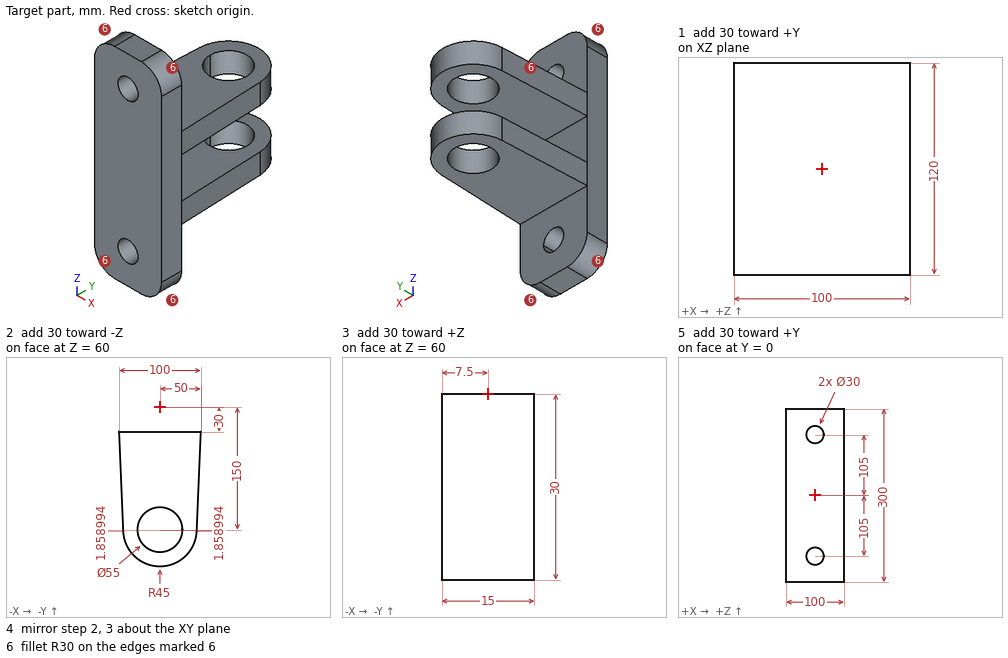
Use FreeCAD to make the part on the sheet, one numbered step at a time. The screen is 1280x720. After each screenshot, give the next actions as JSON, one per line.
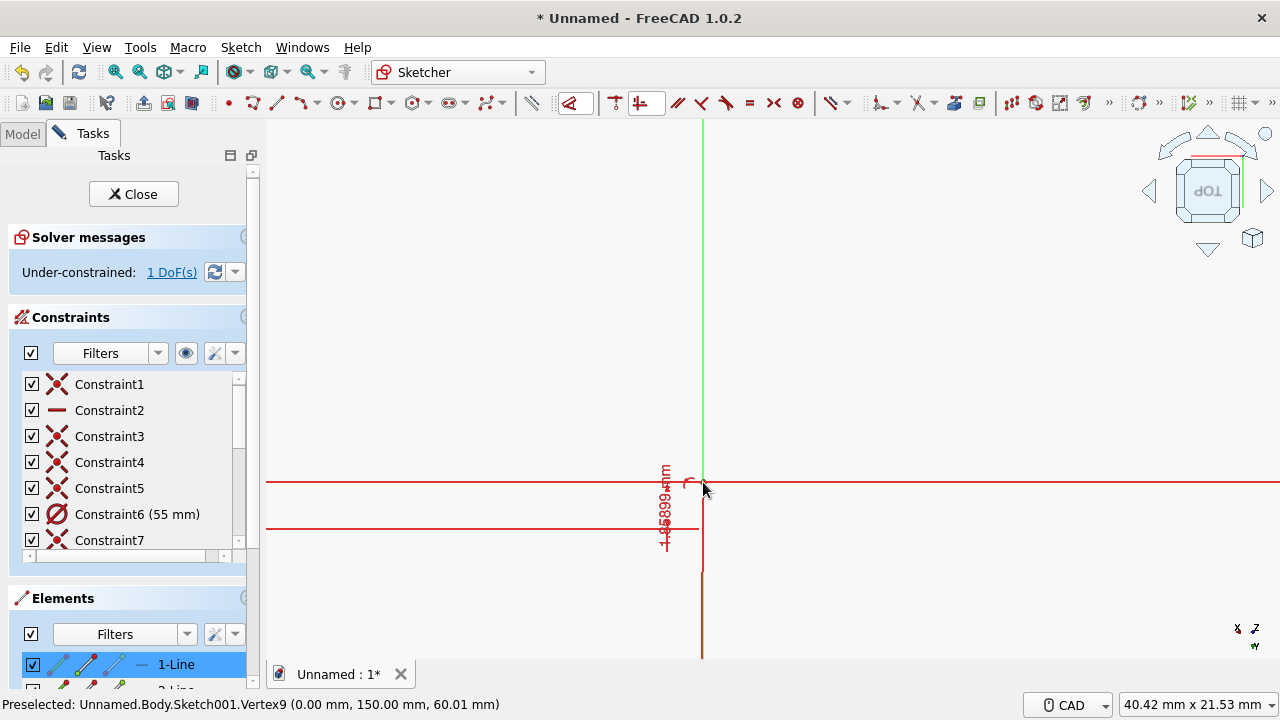
{"action": "key", "text": "i"}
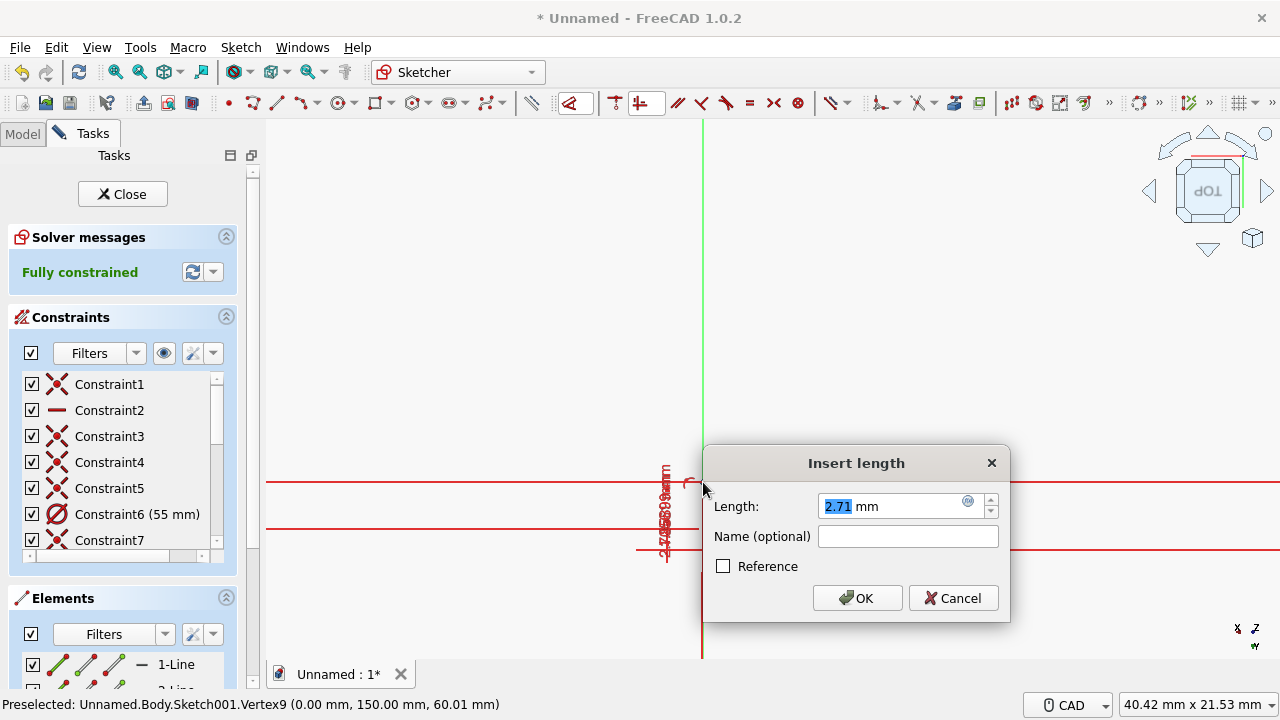
{"action": "type", "text": "1.858994"}
{"action": "key", "text": "Return"}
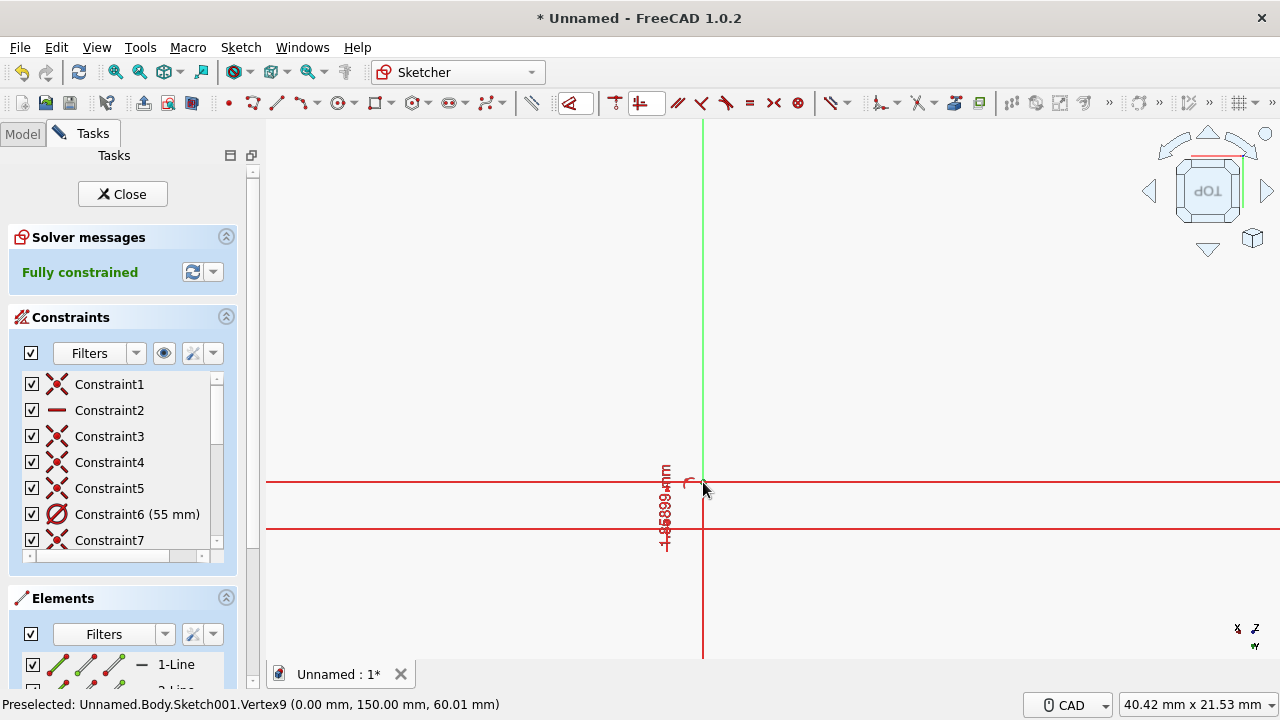
{"action": "left_click", "coordinate": [123, 194]}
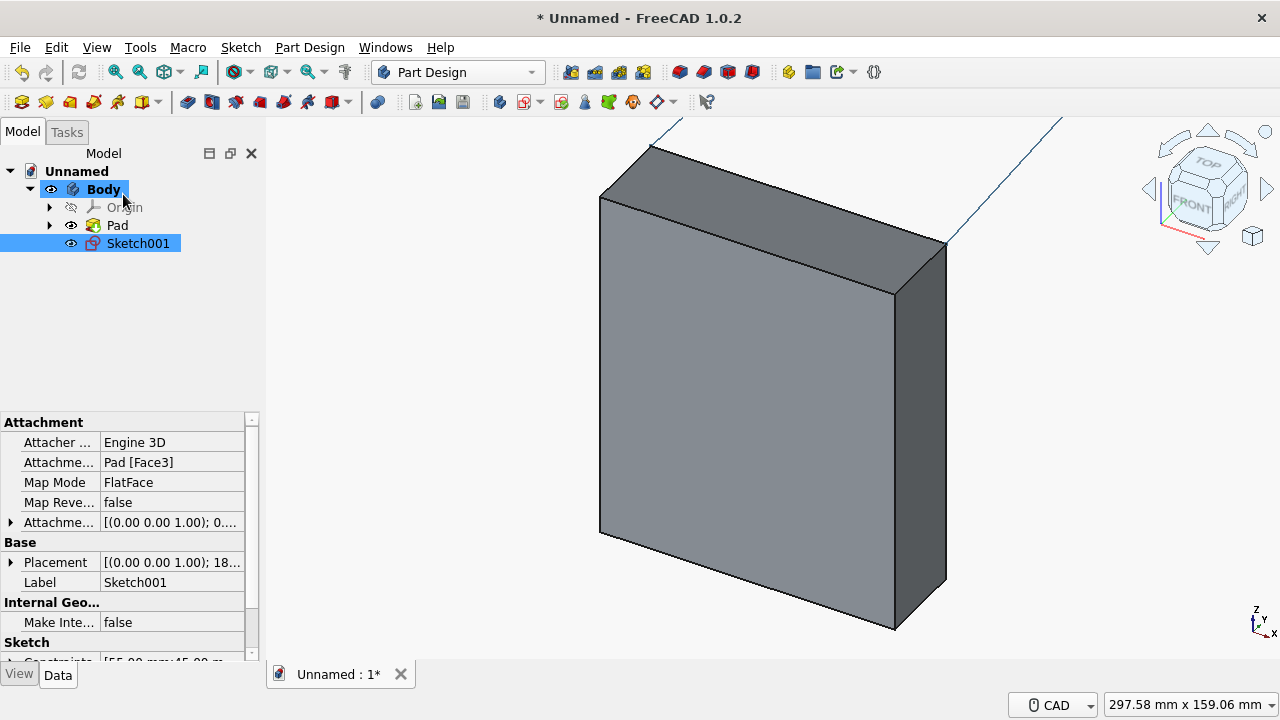
{"action": "left_click", "coordinate": [22, 102]}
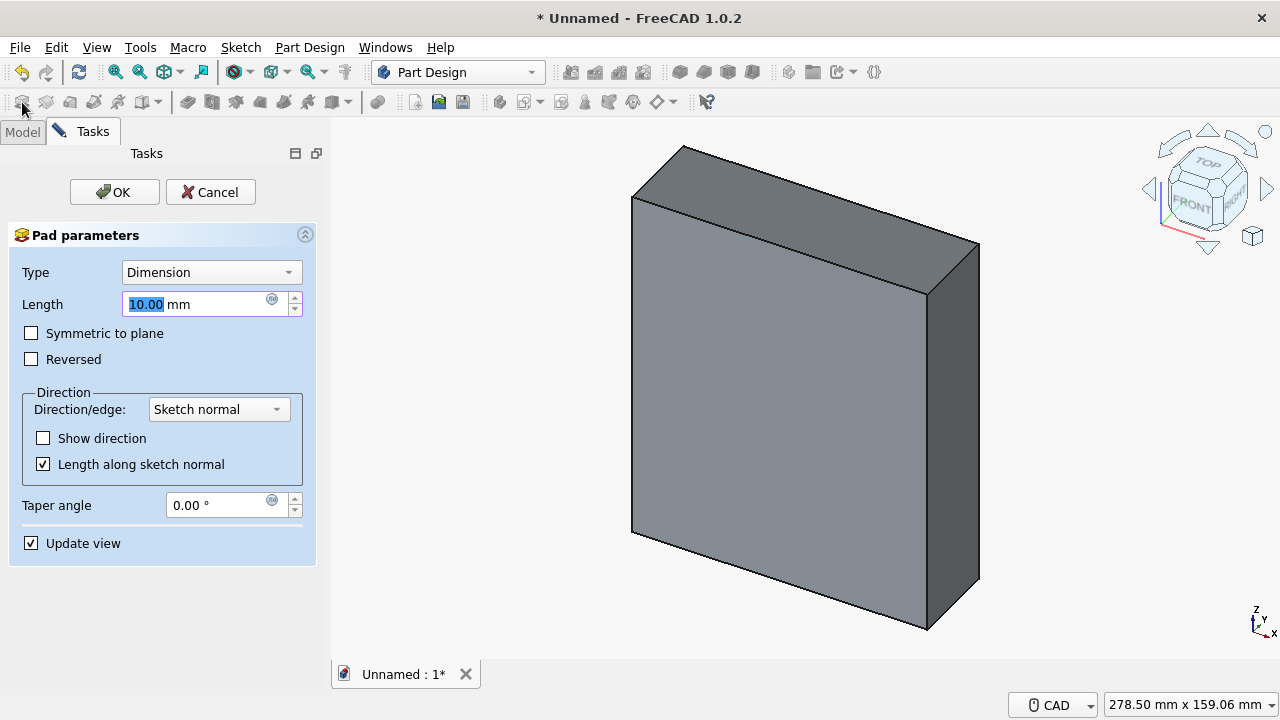
{"action": "type", "text": "30"}
{"action": "key", "text": "Tab"}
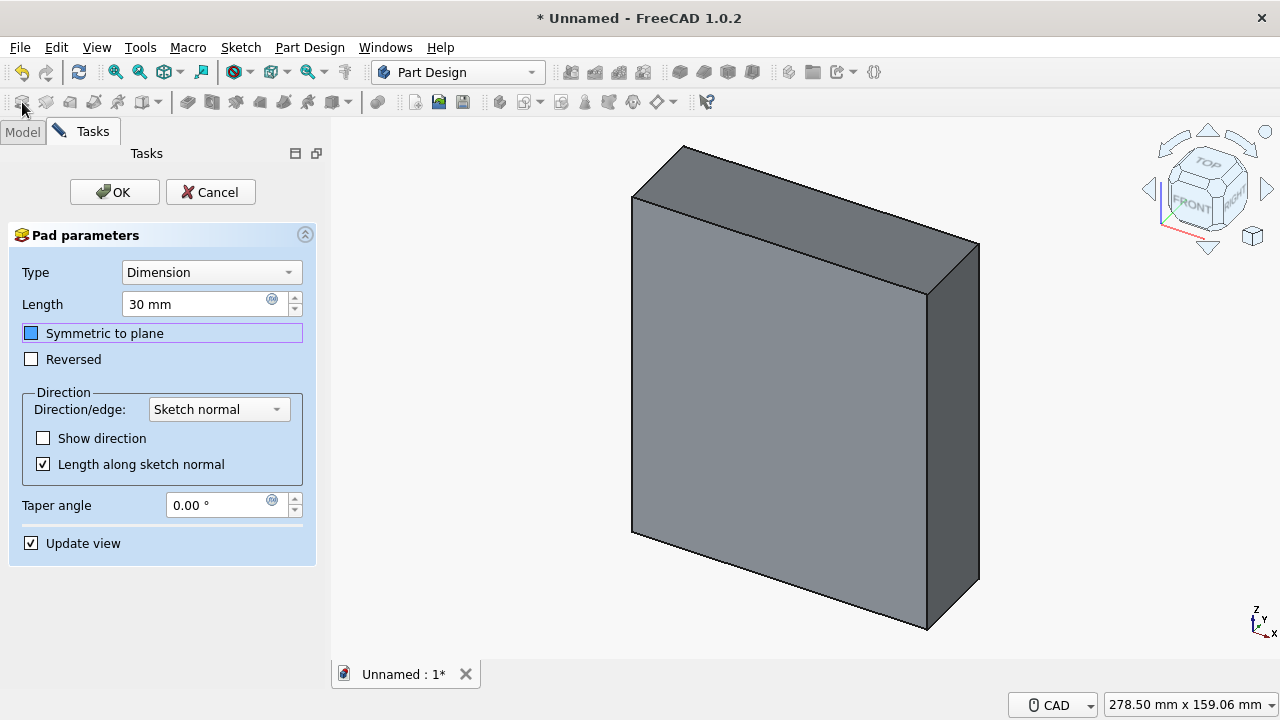
{"action": "left_click", "coordinate": [30, 359]}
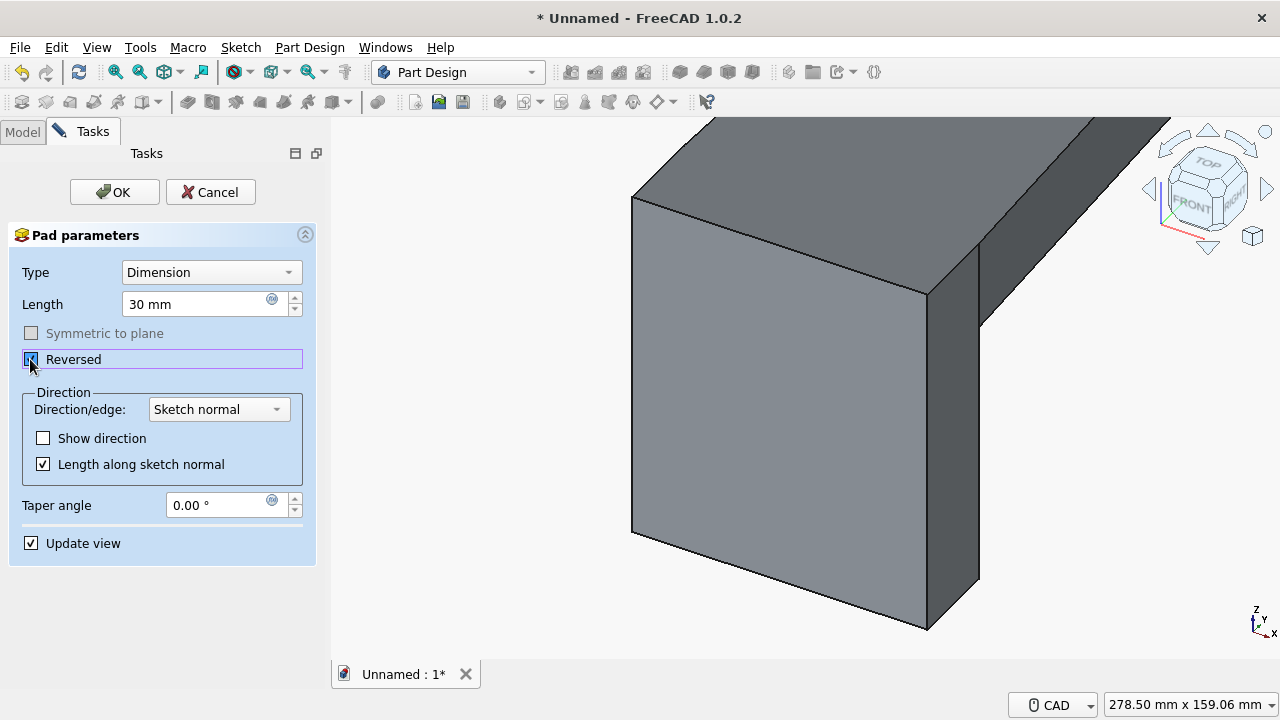
{"action": "left_click", "coordinate": [115, 192]}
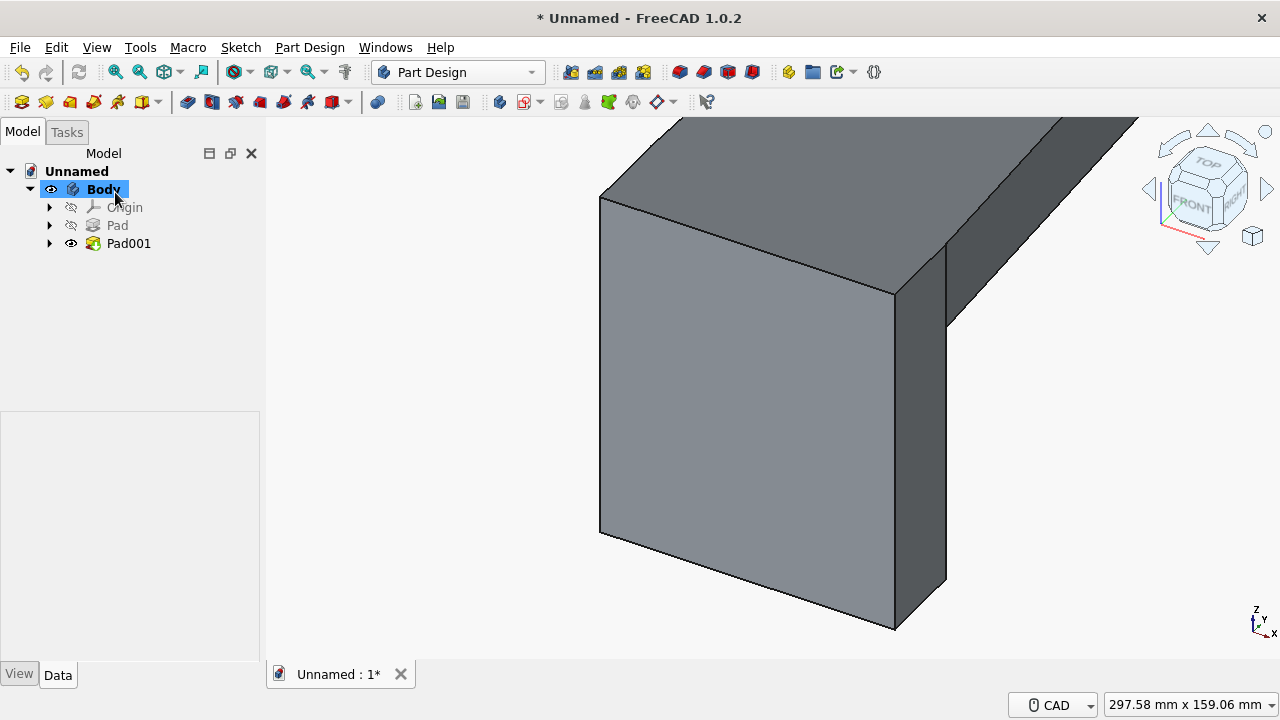
{"action": "left_click", "coordinate": [116, 72]}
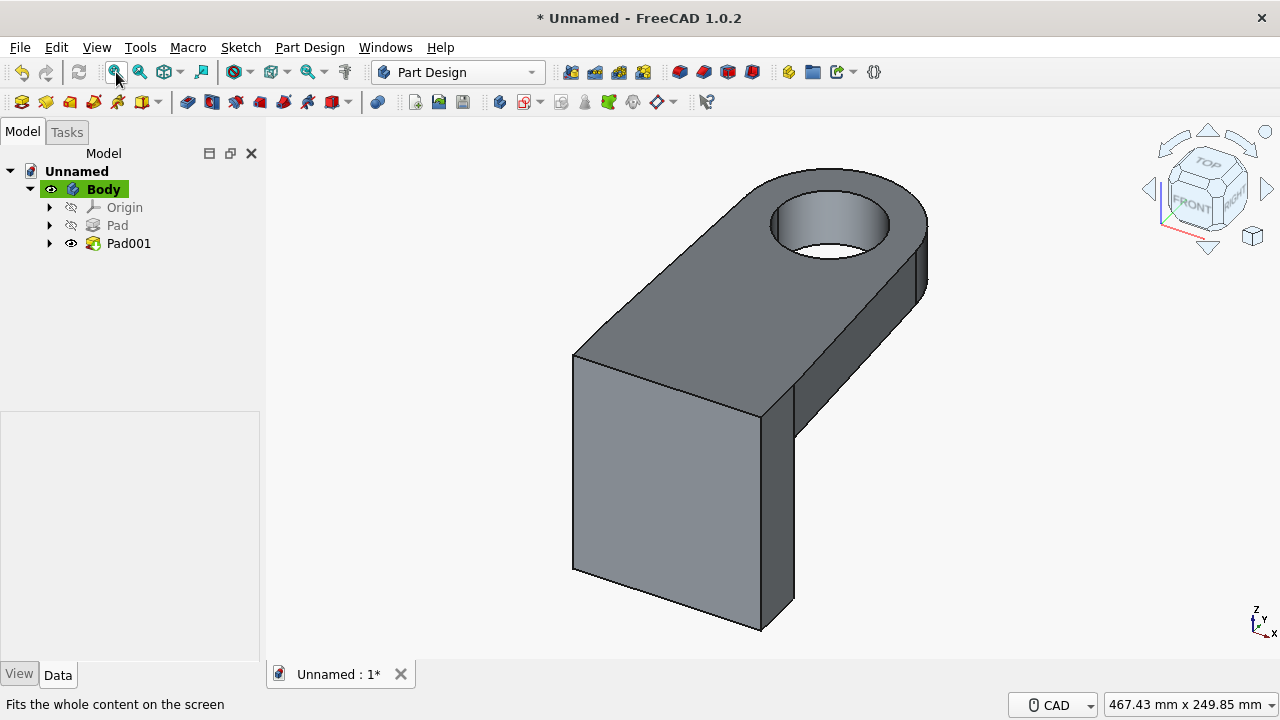
{"action": "left_click", "coordinate": [743, 310]}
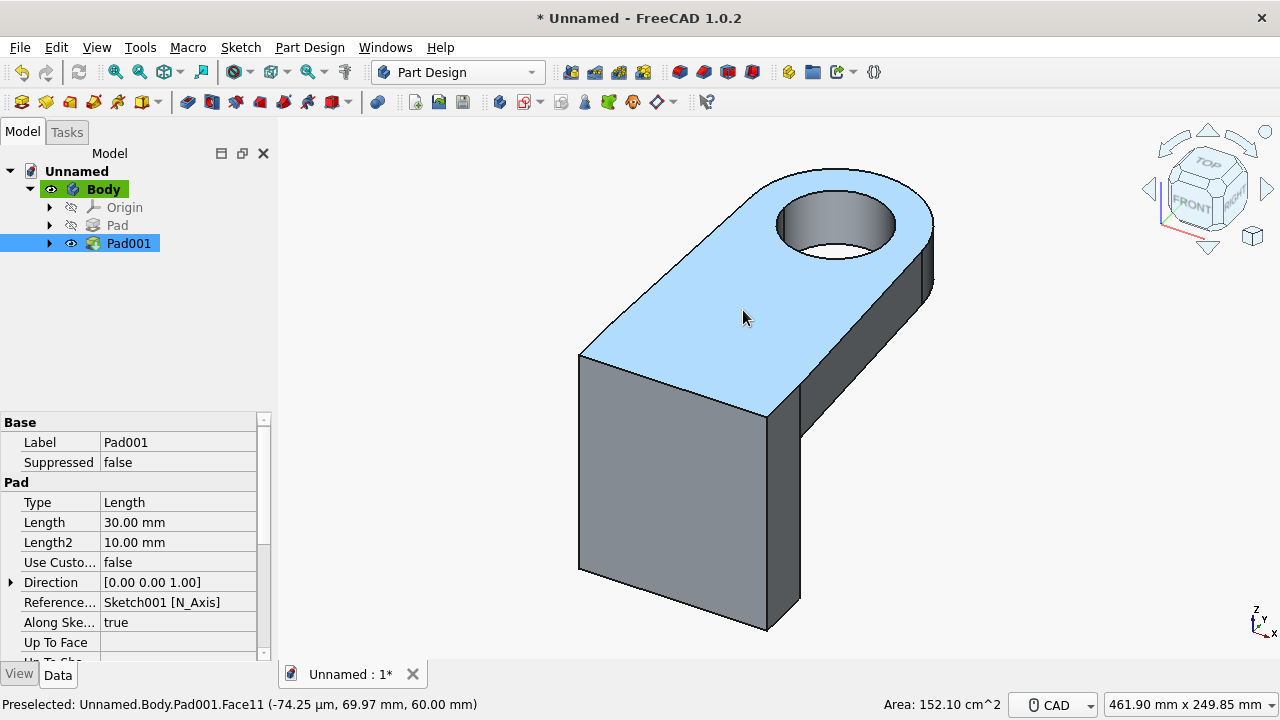
{"action": "left_click", "coordinate": [524, 102]}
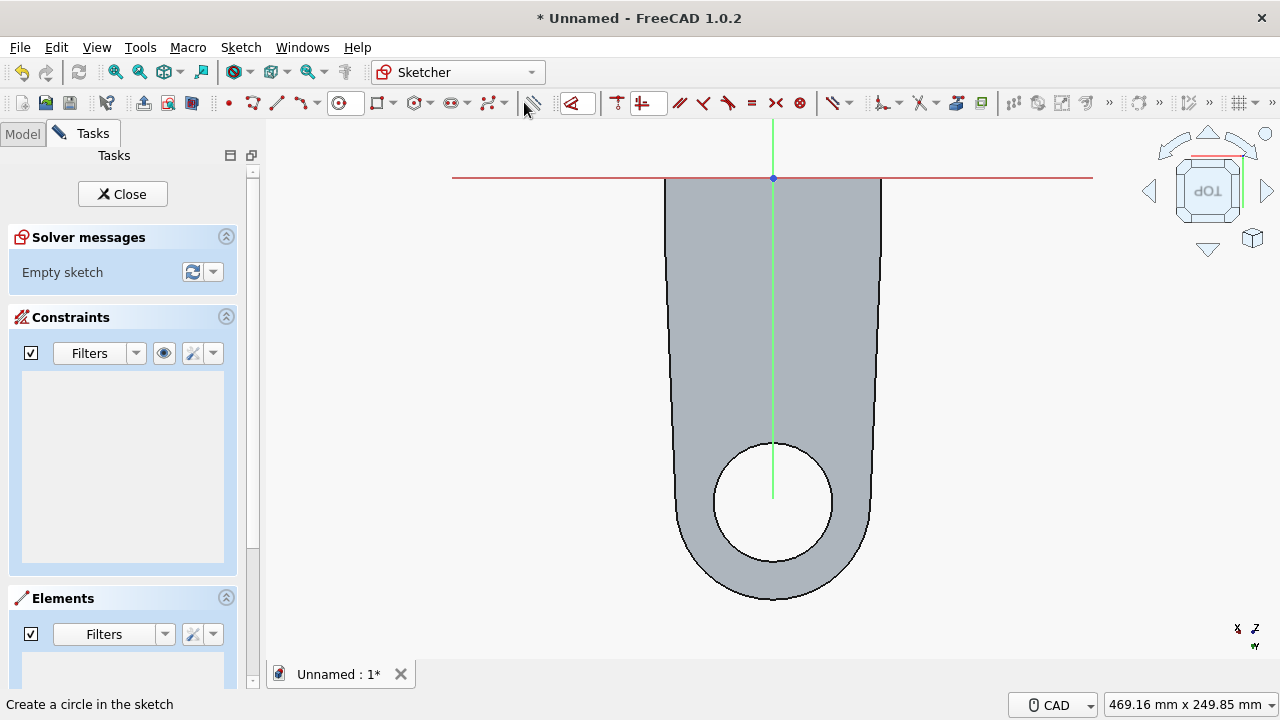
{"action": "scroll", "coordinate": [790, 166], "scroll_direction": "up", "scroll_amount": 8}